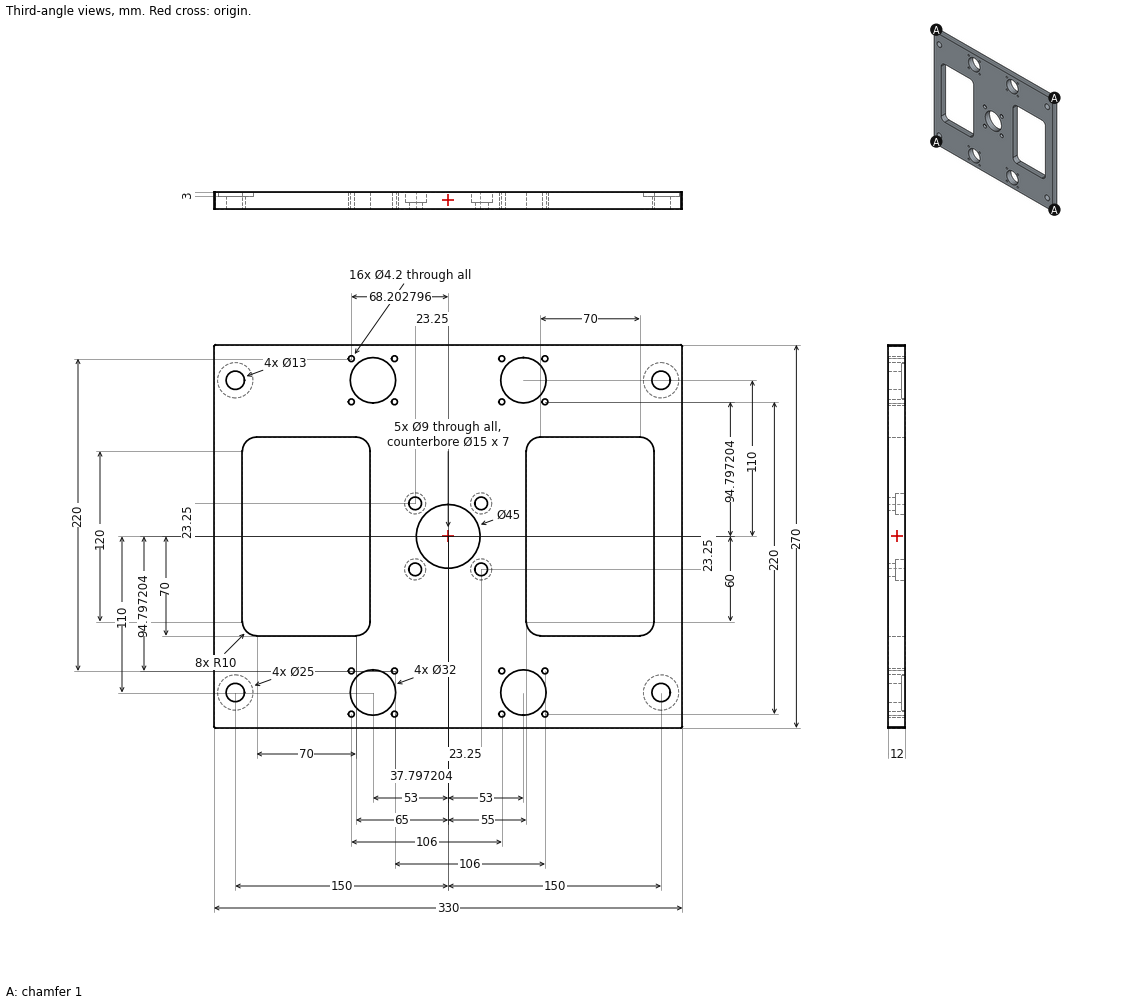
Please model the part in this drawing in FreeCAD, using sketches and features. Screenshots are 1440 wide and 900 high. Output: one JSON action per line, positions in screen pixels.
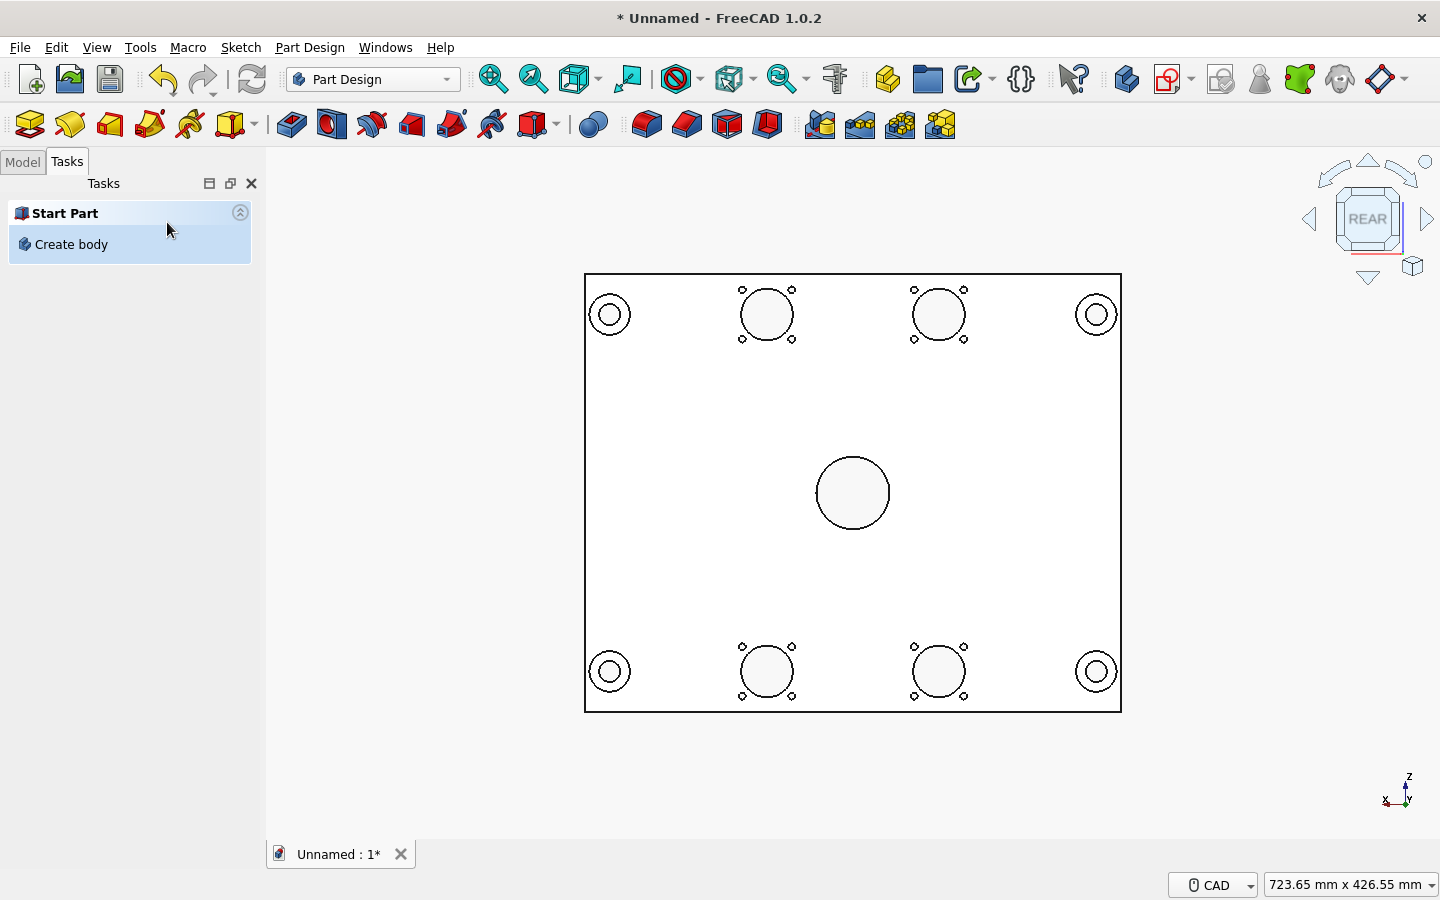
{"action": "left_click", "coordinate": [700, 492]}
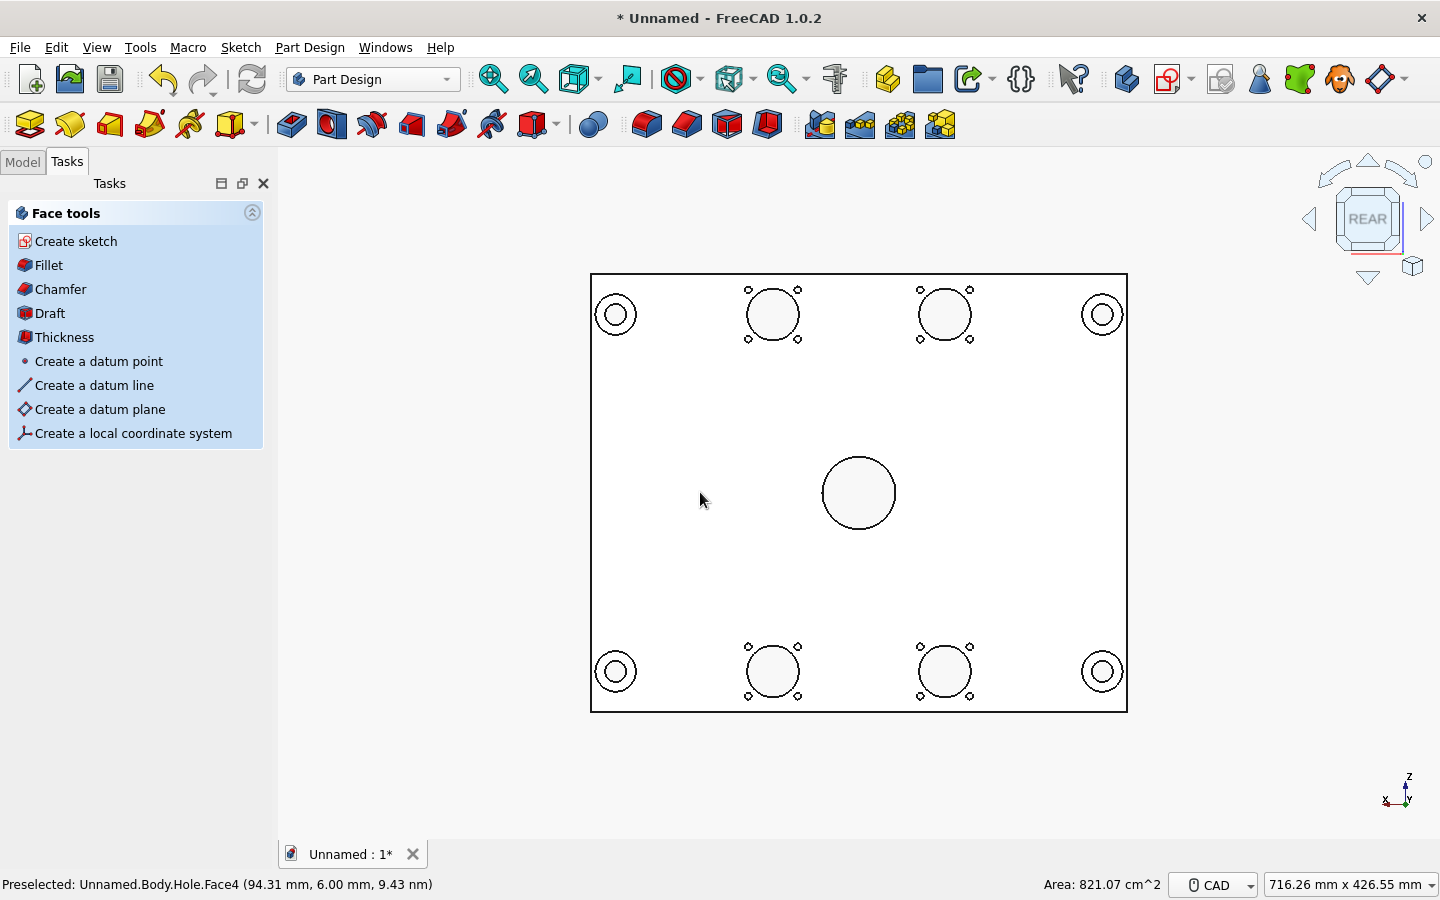
{"action": "left_click", "coordinate": [1168, 80]}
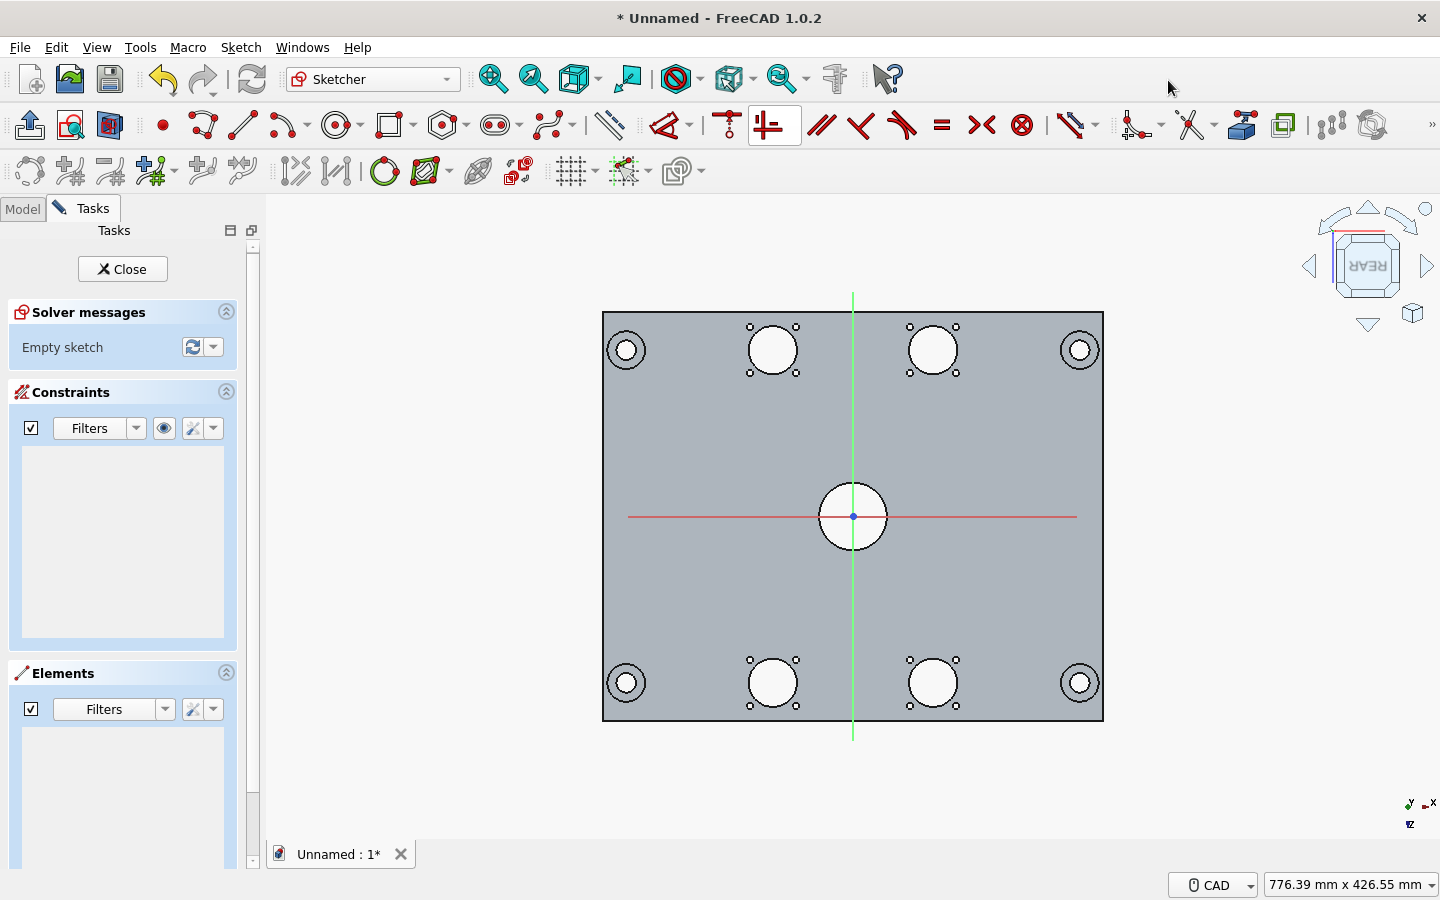
{"action": "scroll", "coordinate": [870, 516], "scroll_direction": "up", "scroll_amount": 8}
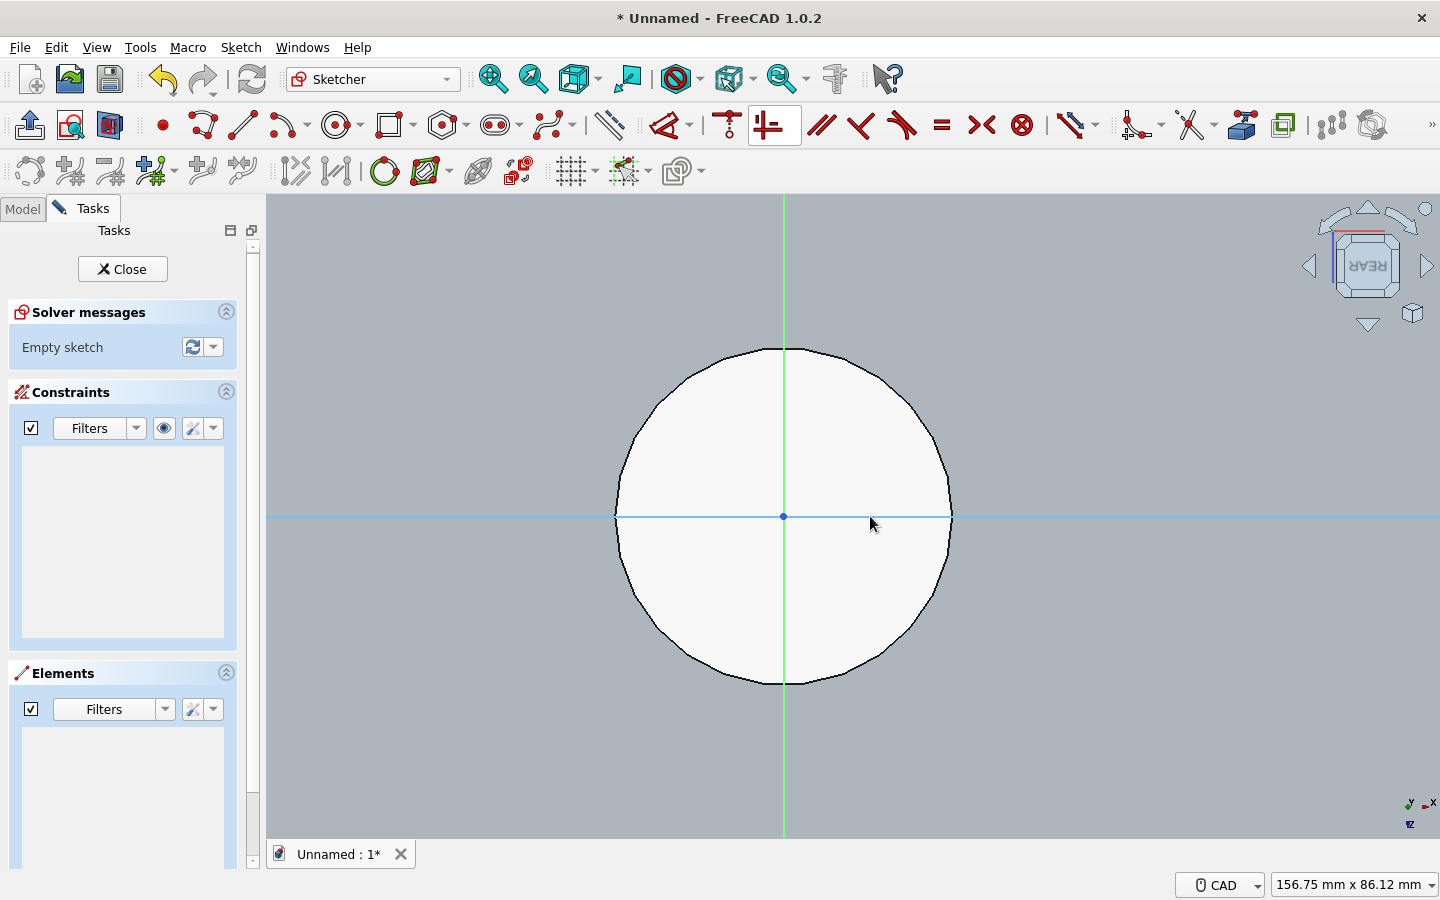
{"action": "key", "text": "g c"}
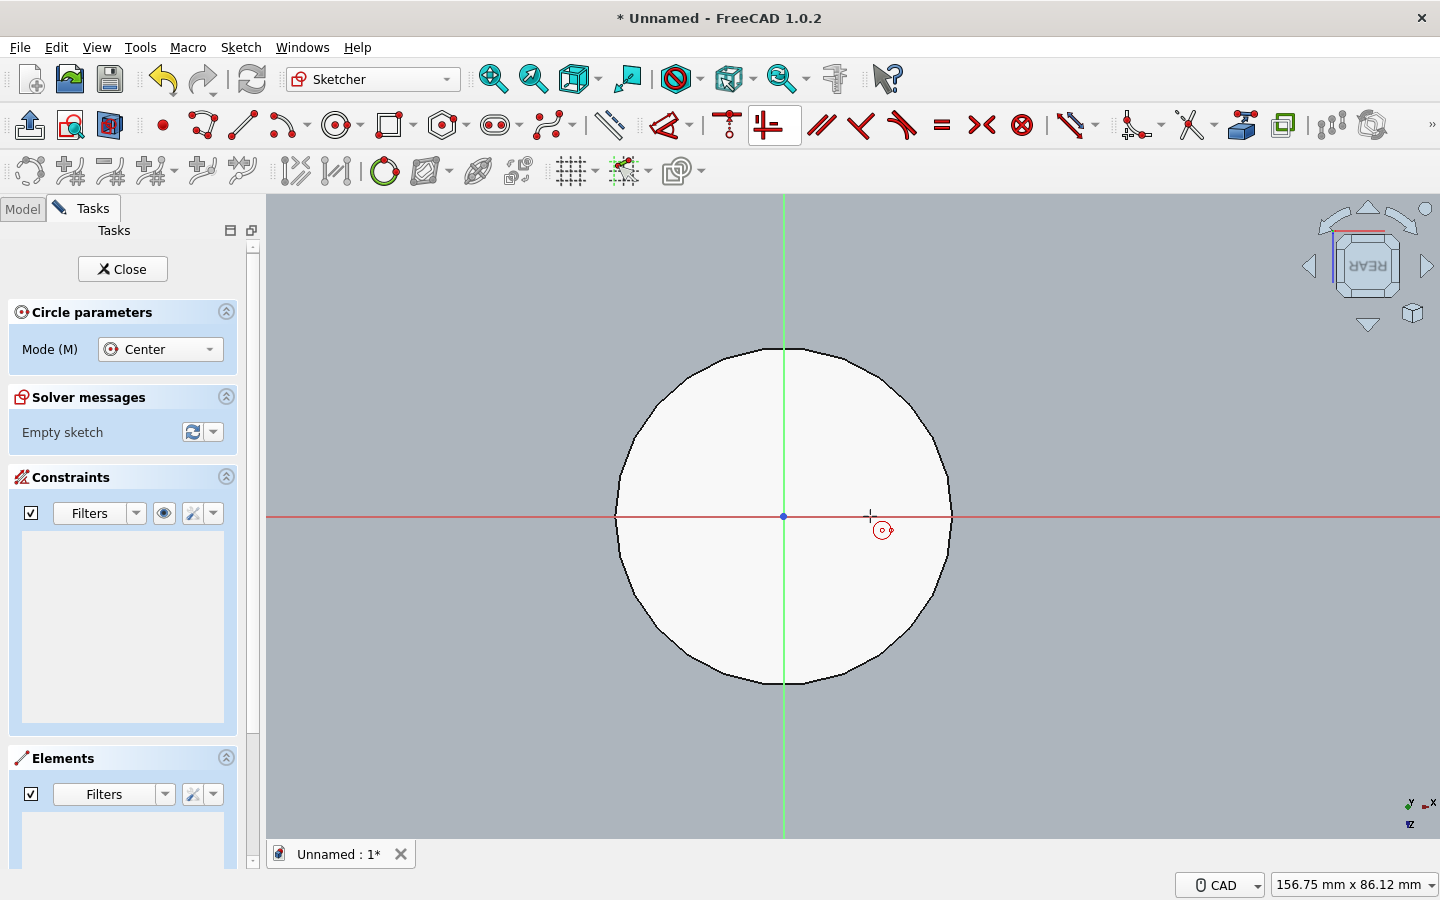
{"action": "left_click", "coordinate": [784, 516]}
{"action": "mouse_move", "coordinate": [808, 493]}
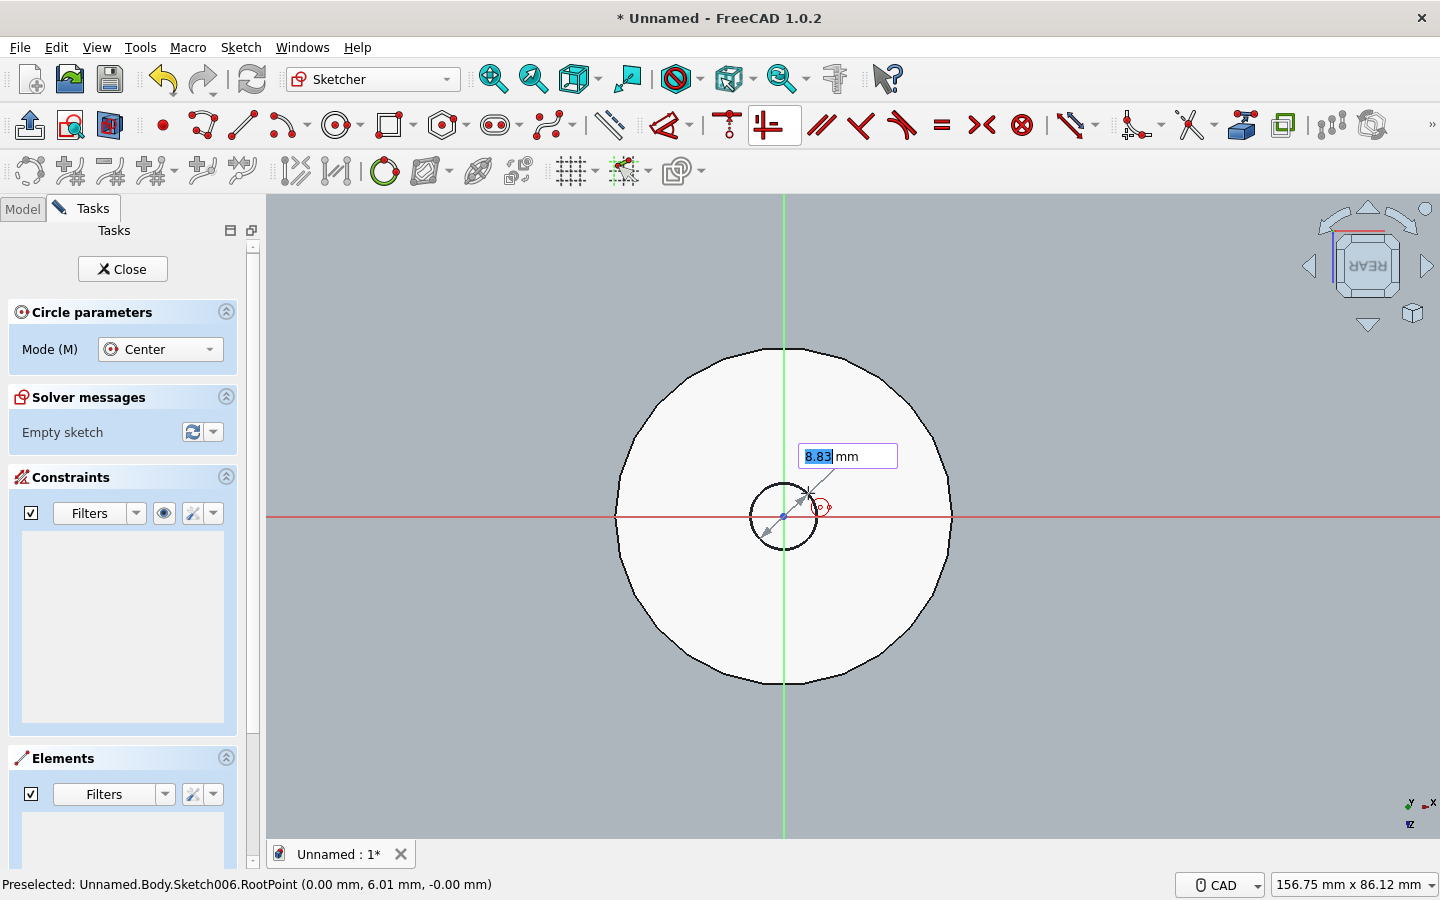
{"action": "type", "text": "9"}
{"action": "key", "text": "Return"}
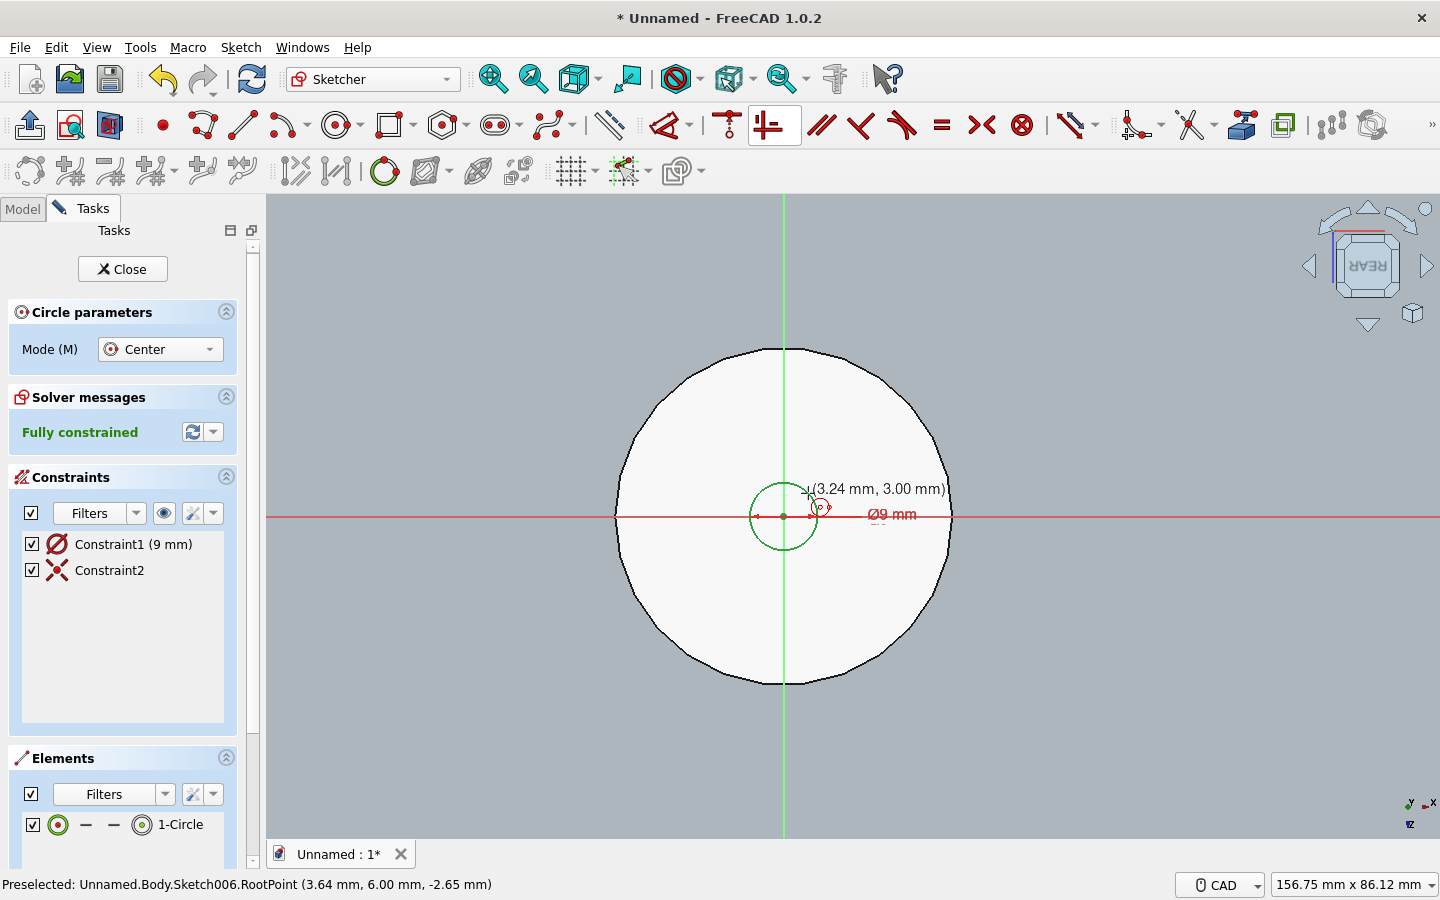
{"action": "left_click", "coordinate": [958, 342]}
{"action": "mouse_move", "coordinate": [982, 319]}